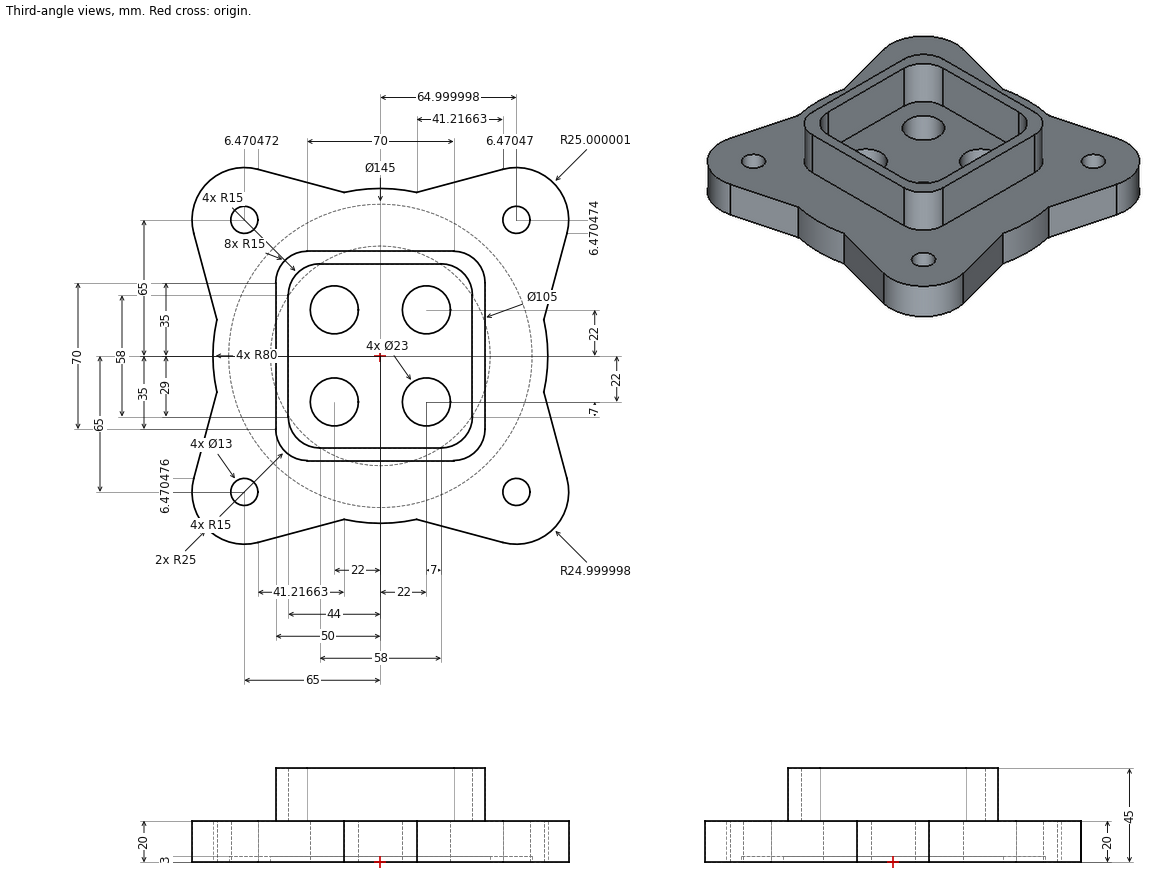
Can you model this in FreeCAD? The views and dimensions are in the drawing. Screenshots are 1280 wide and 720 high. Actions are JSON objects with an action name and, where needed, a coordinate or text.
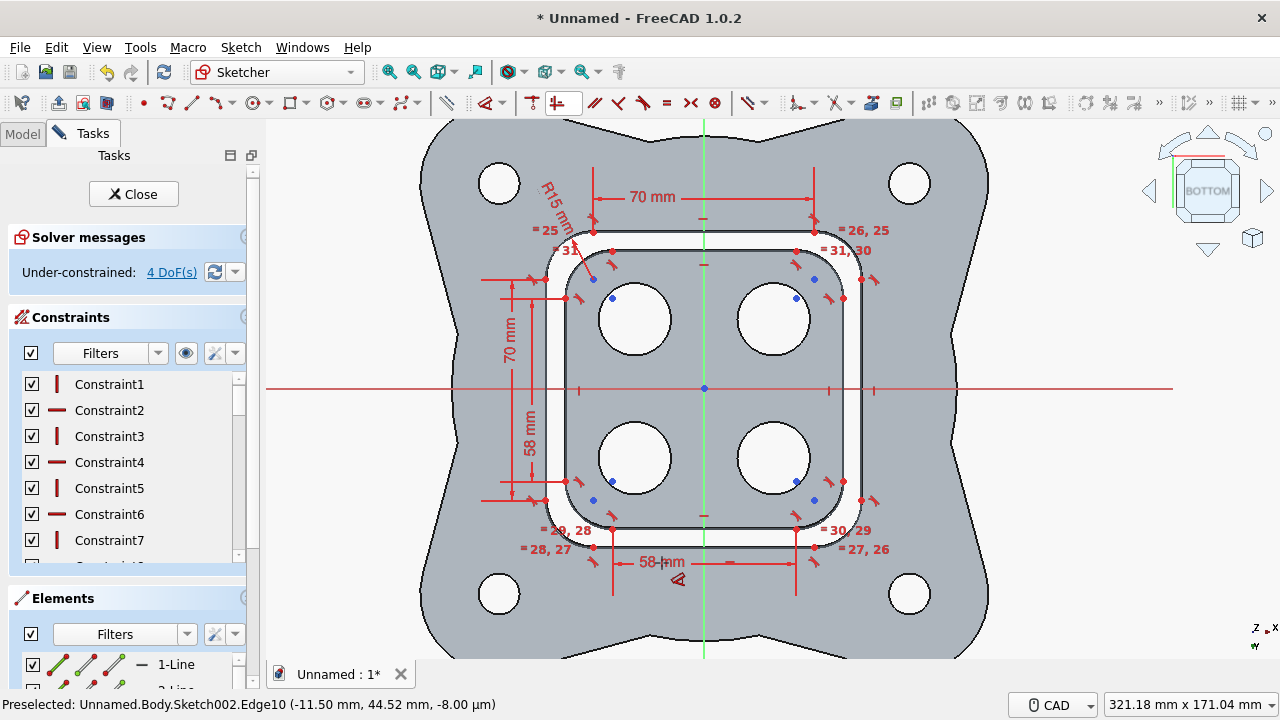
{"action": "left_click", "coordinate": [546, 501]}
{"action": "left_click", "coordinate": [625, 355]}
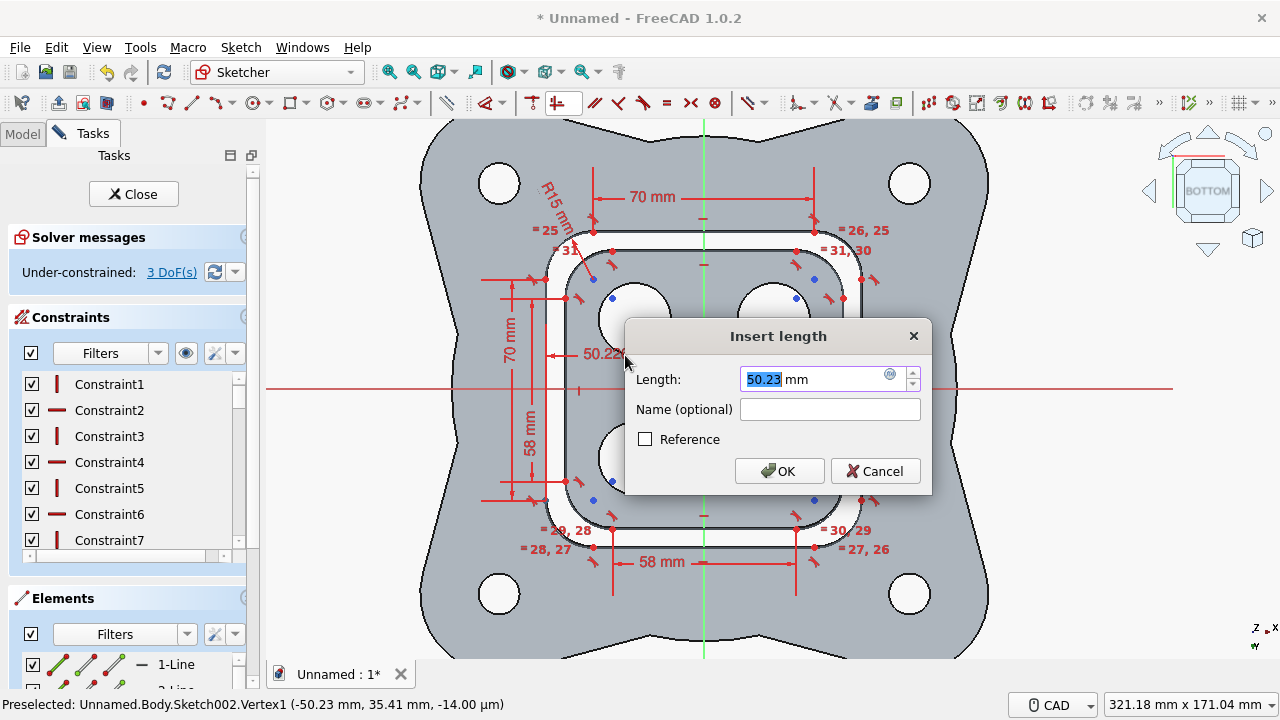
{"action": "type", "text": "50"}
{"action": "key", "text": "Return"}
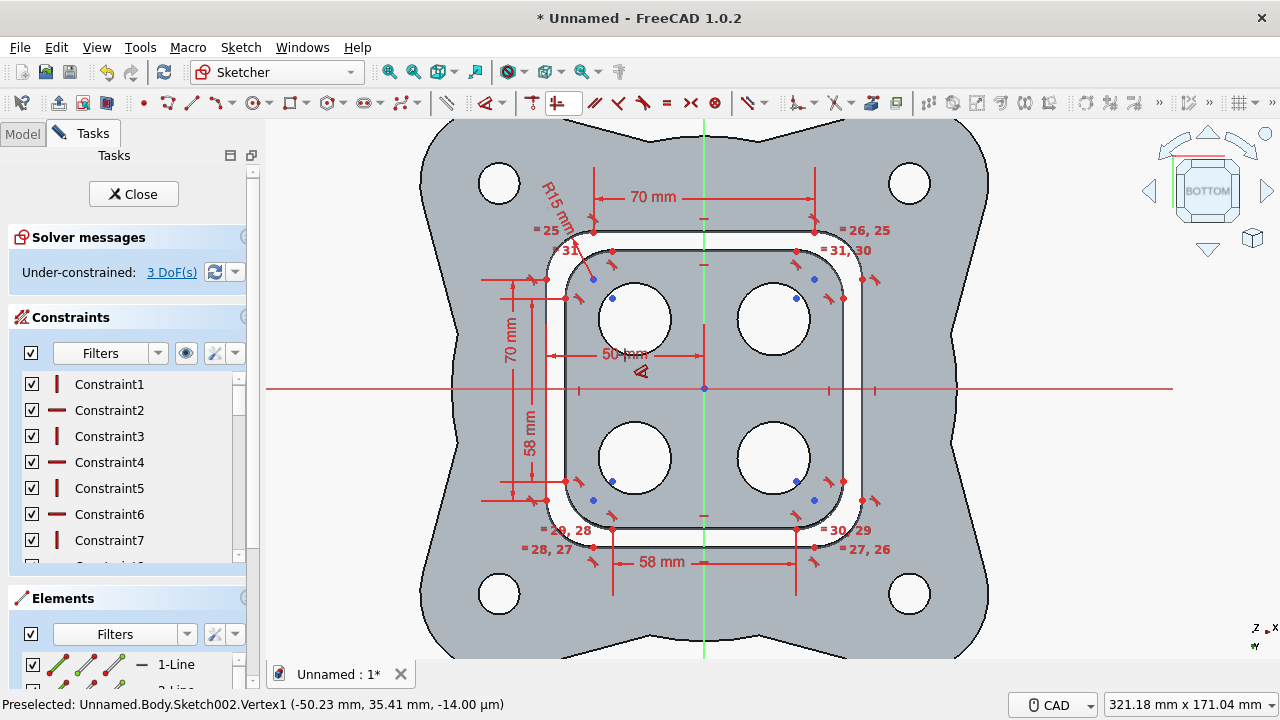
{"action": "left_click", "coordinate": [546, 501]}
{"action": "left_click", "coordinate": [512, 470]}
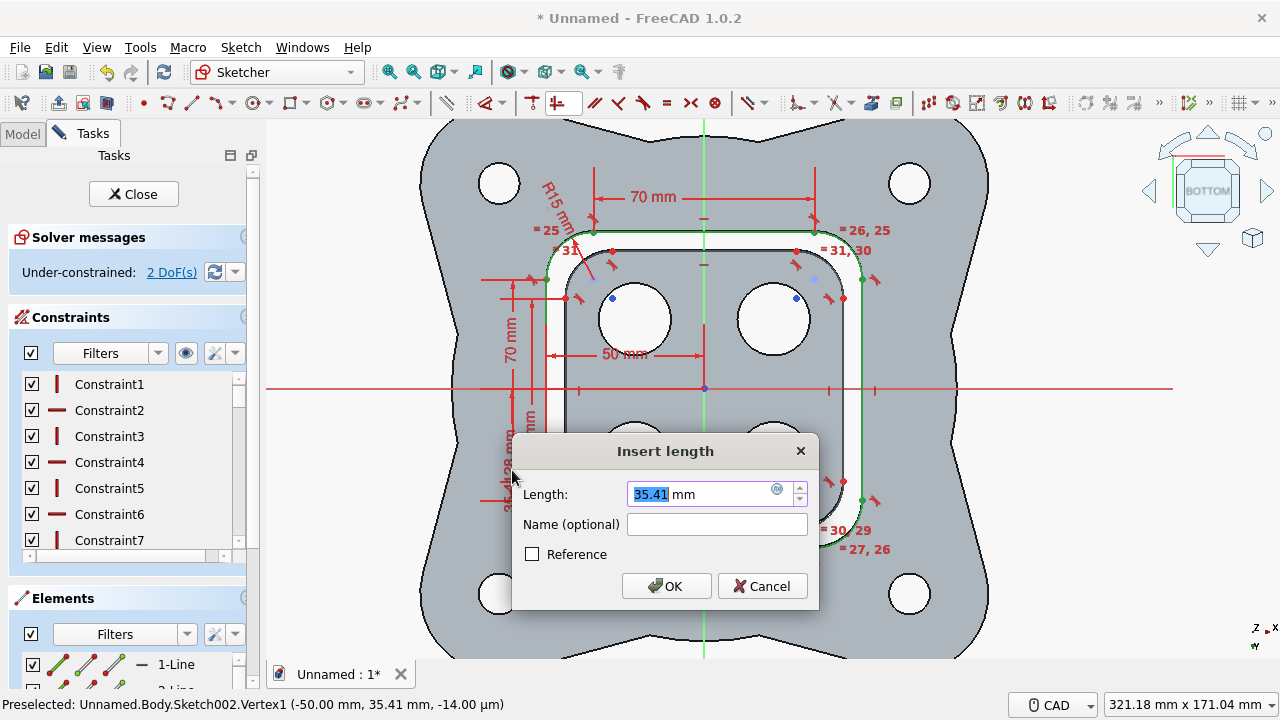
{"action": "type", "text": "35"}
{"action": "key", "text": "Return"}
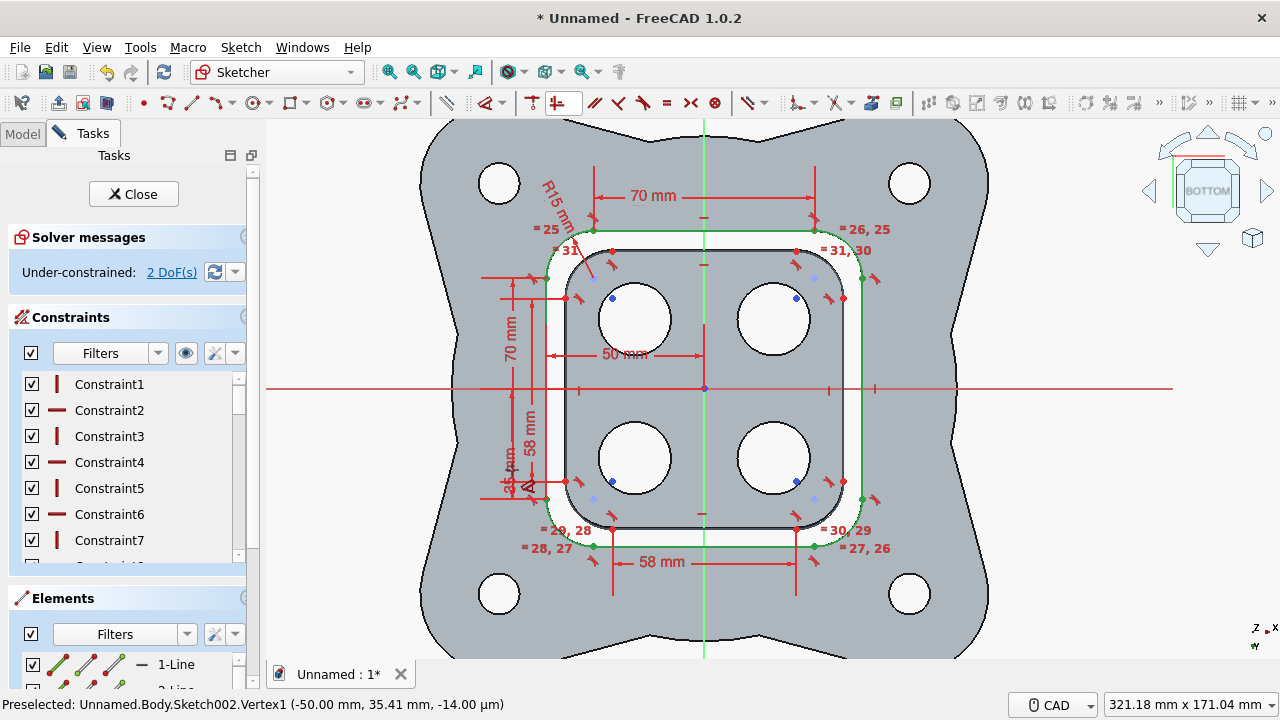
{"action": "left_click", "coordinate": [566, 299]}
{"action": "left_click", "coordinate": [635, 265]}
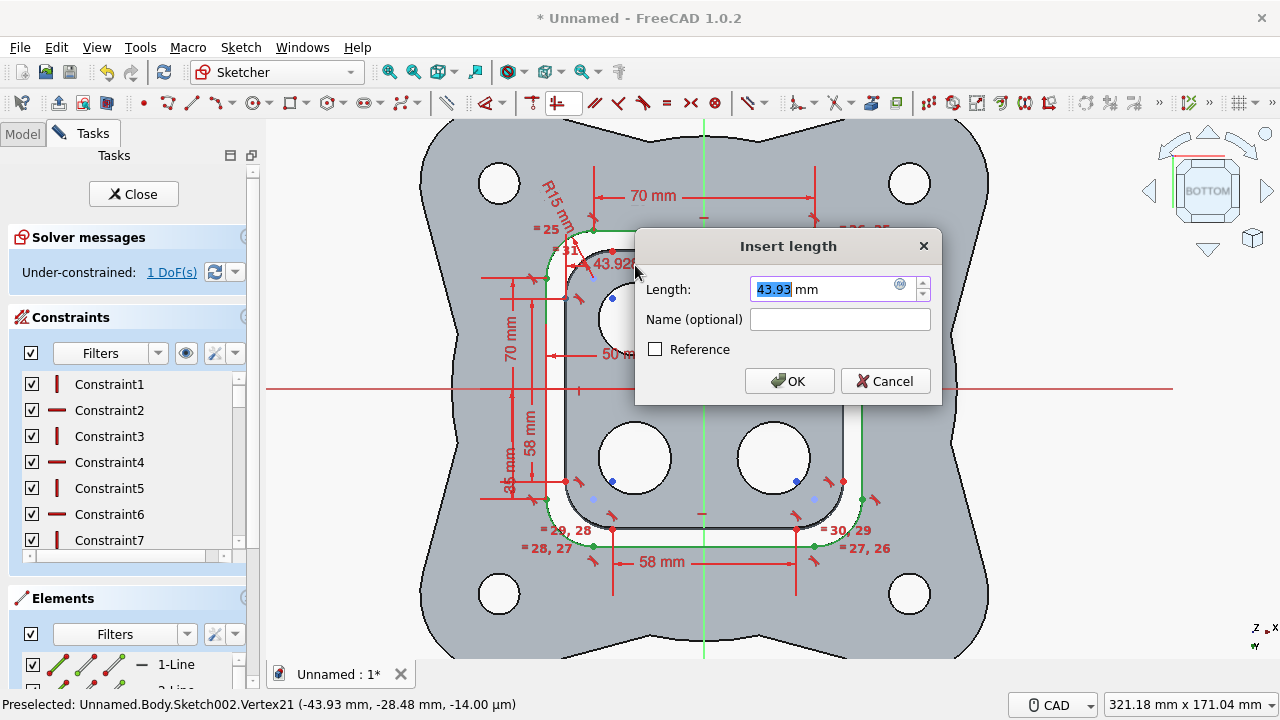
{"action": "type", "text": "44"}
{"action": "key", "text": "Return"}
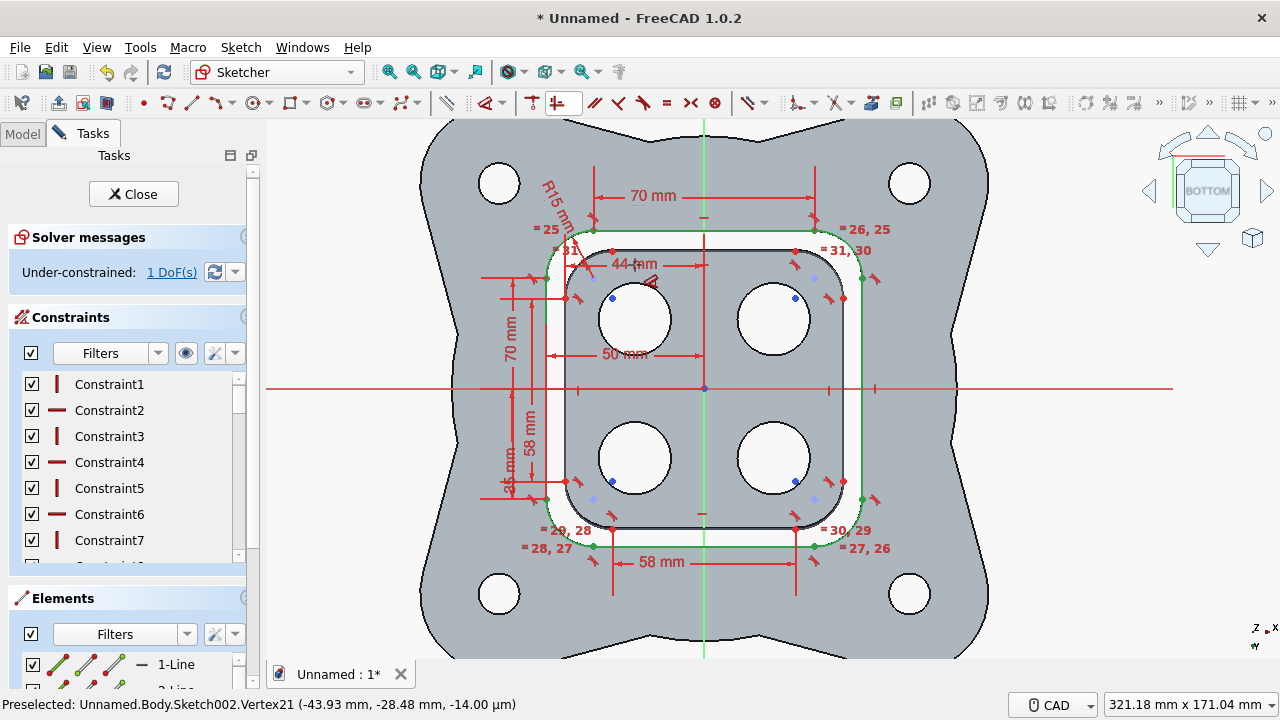
{"action": "left_click", "coordinate": [565, 299]}
{"action": "left_click", "coordinate": [531, 364]}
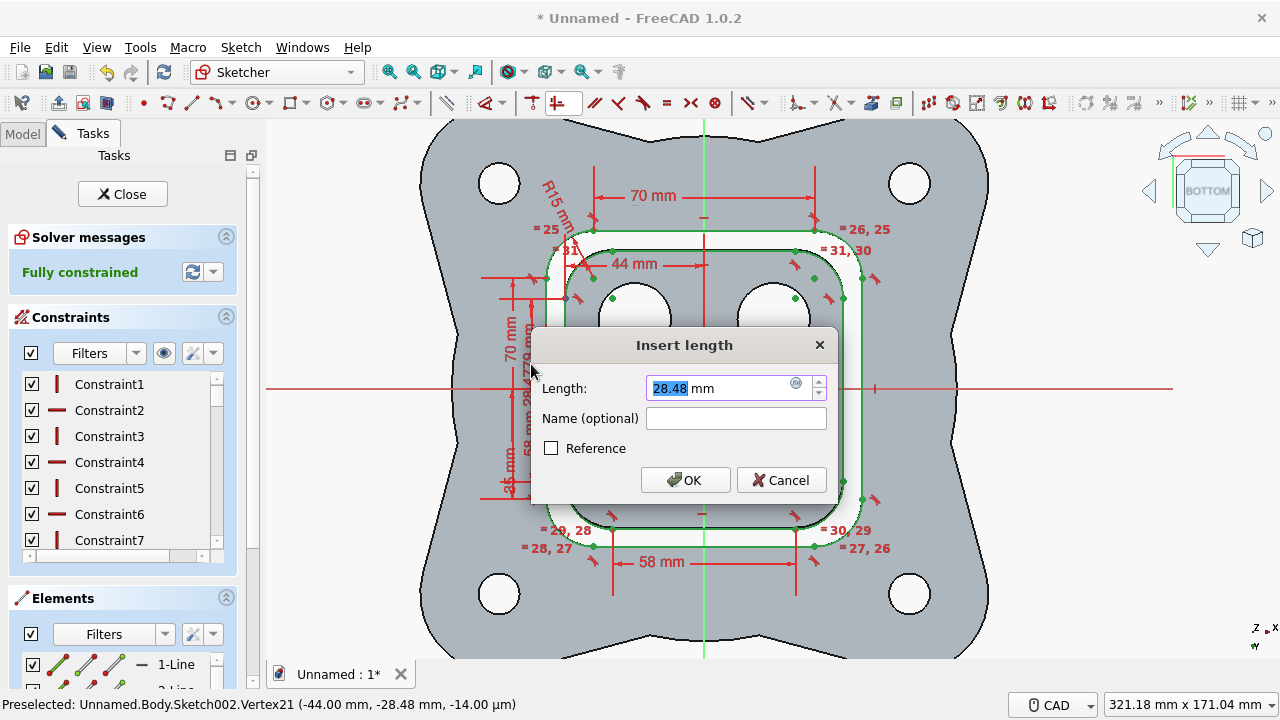
{"action": "type", "text": "29"}
{"action": "key", "text": "Return"}
{"action": "key", "text": "Escape"}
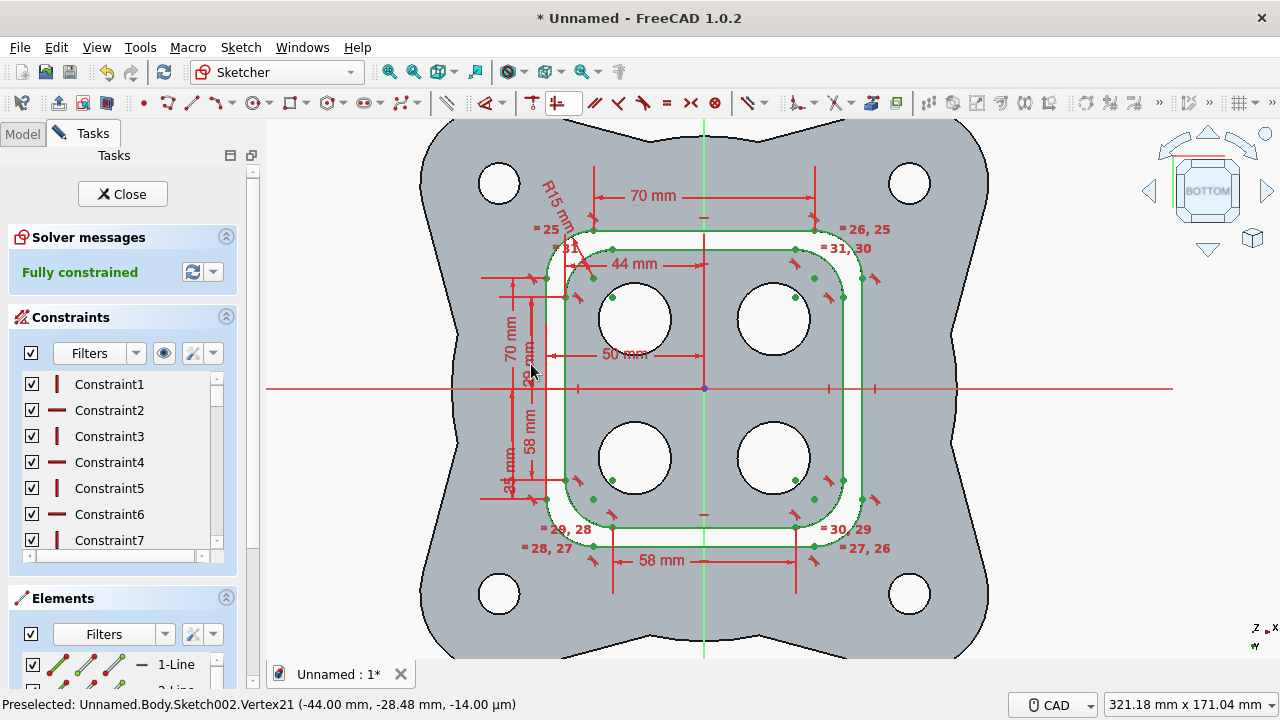
{"action": "left_click", "coordinate": [123, 194]}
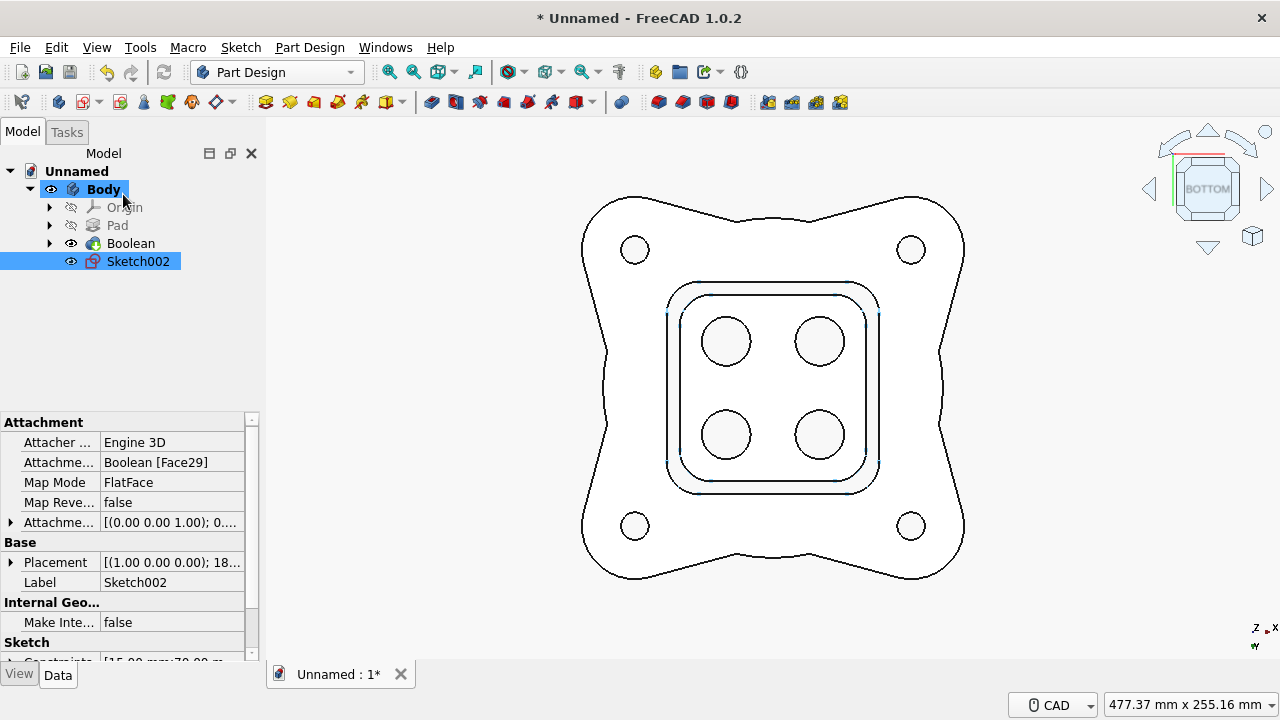
{"action": "left_click", "coordinate": [266, 102]}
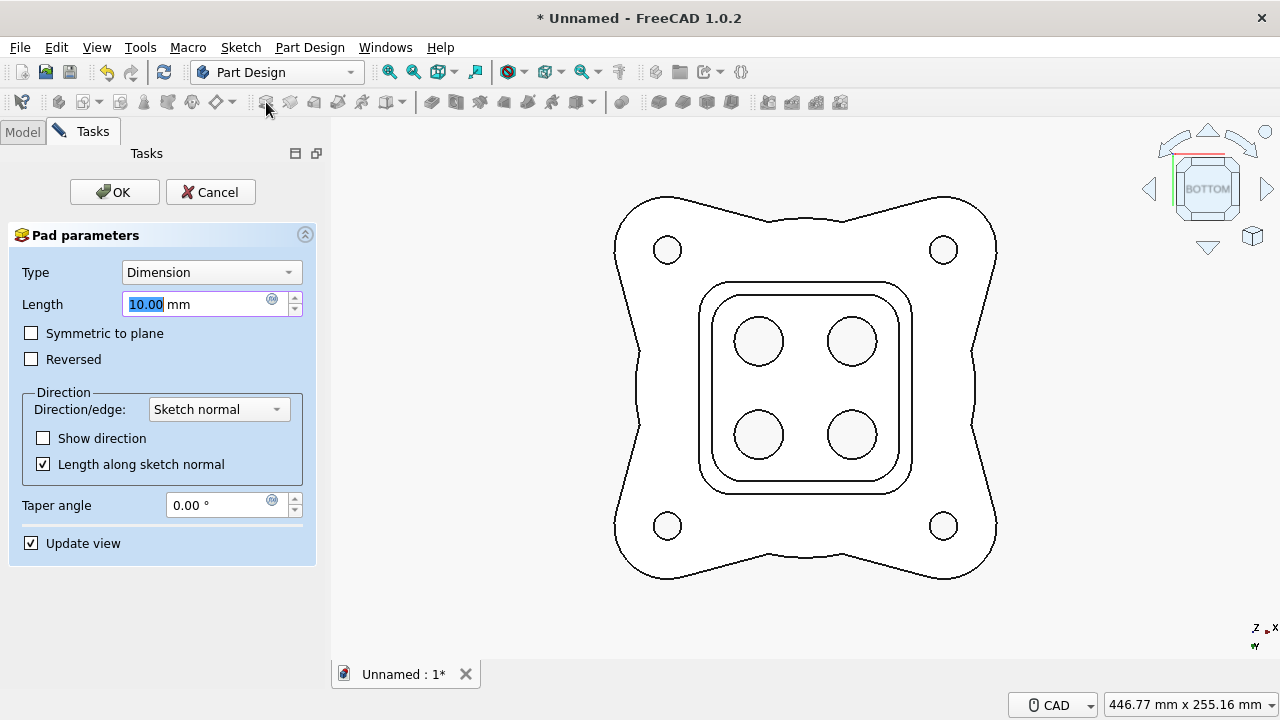
{"action": "type", "text": "45"}
{"action": "key", "text": "Tab"}